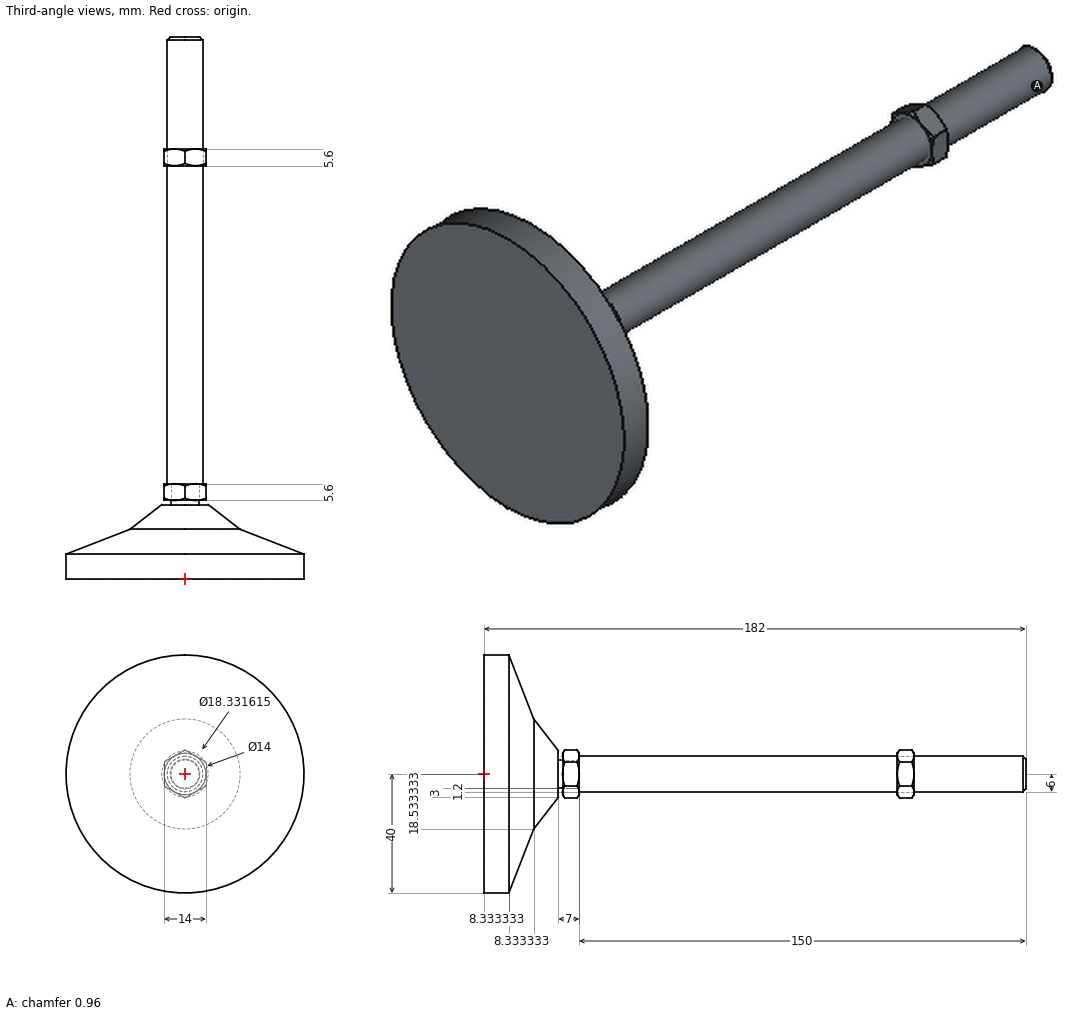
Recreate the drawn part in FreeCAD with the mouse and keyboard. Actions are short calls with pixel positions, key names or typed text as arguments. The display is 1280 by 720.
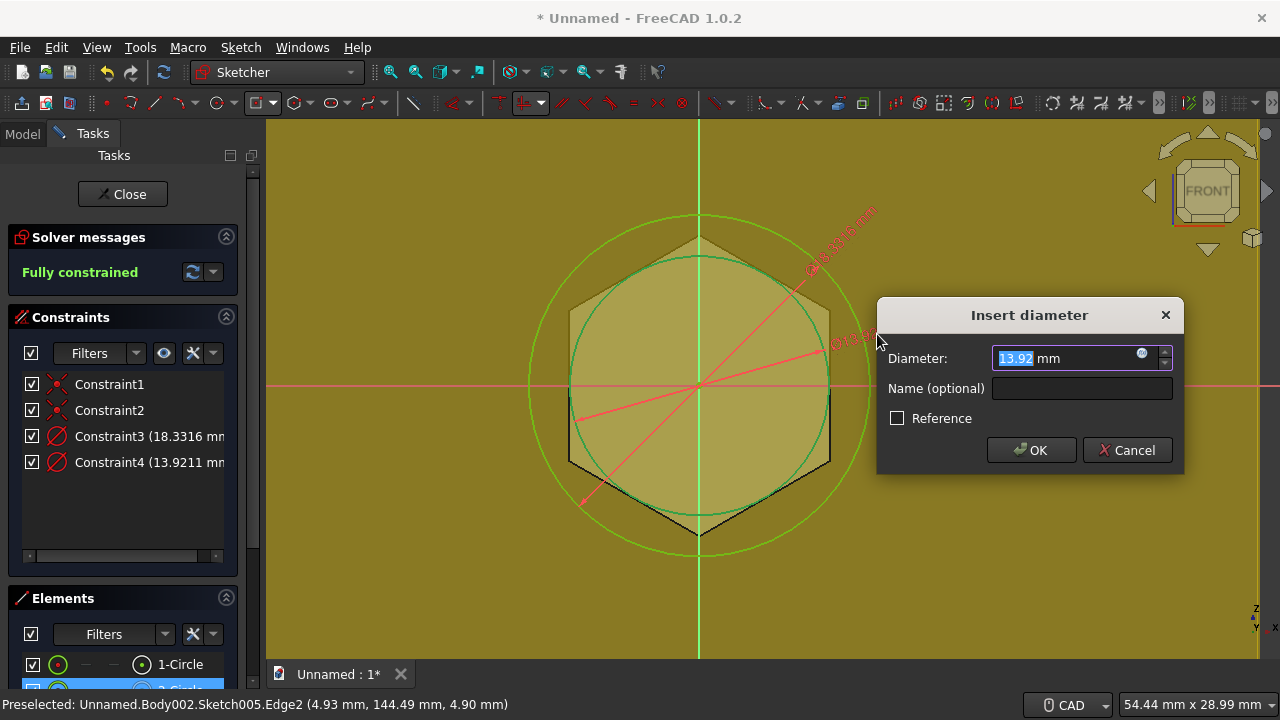
text(14)
key(Return)
key(Escape)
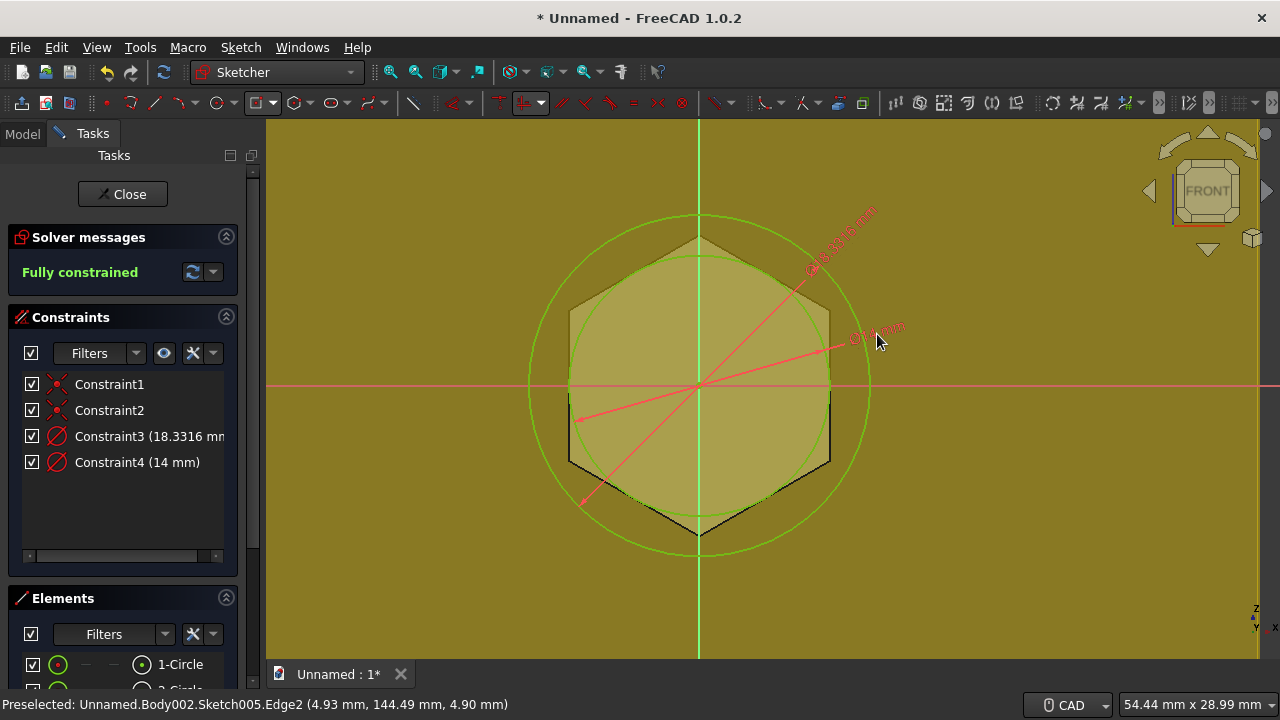
click(123, 194)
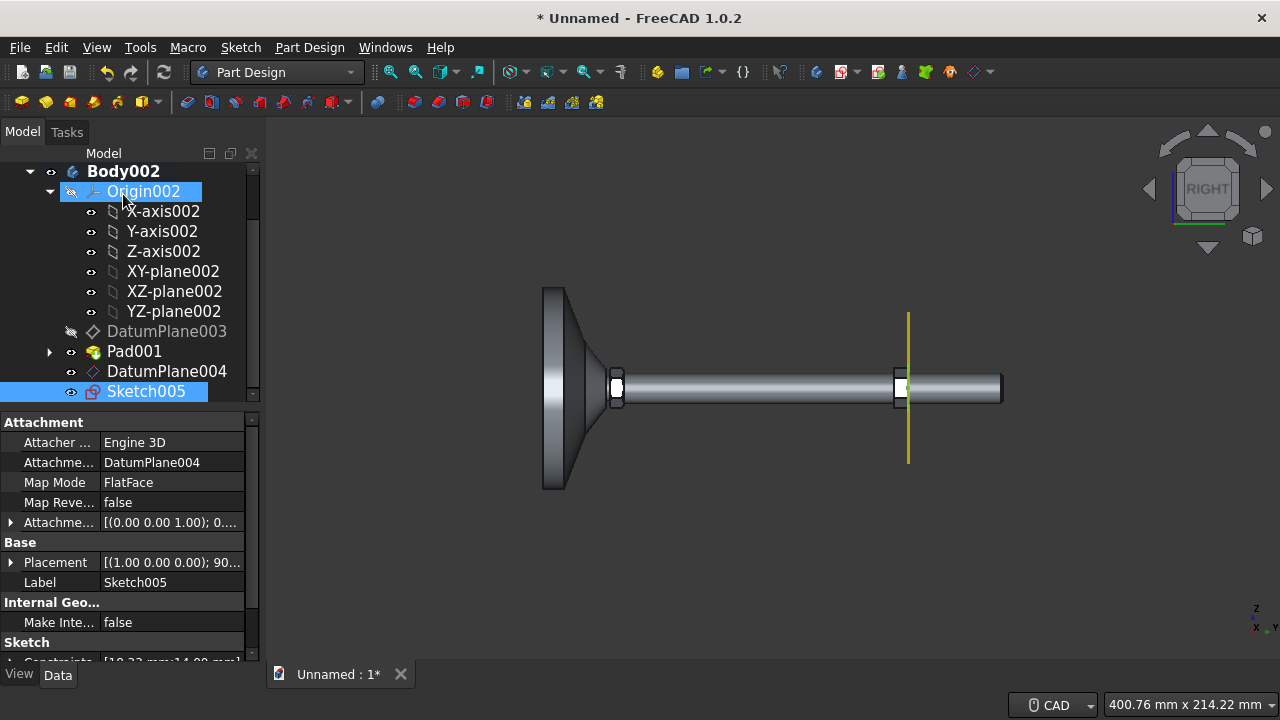
click(188, 102)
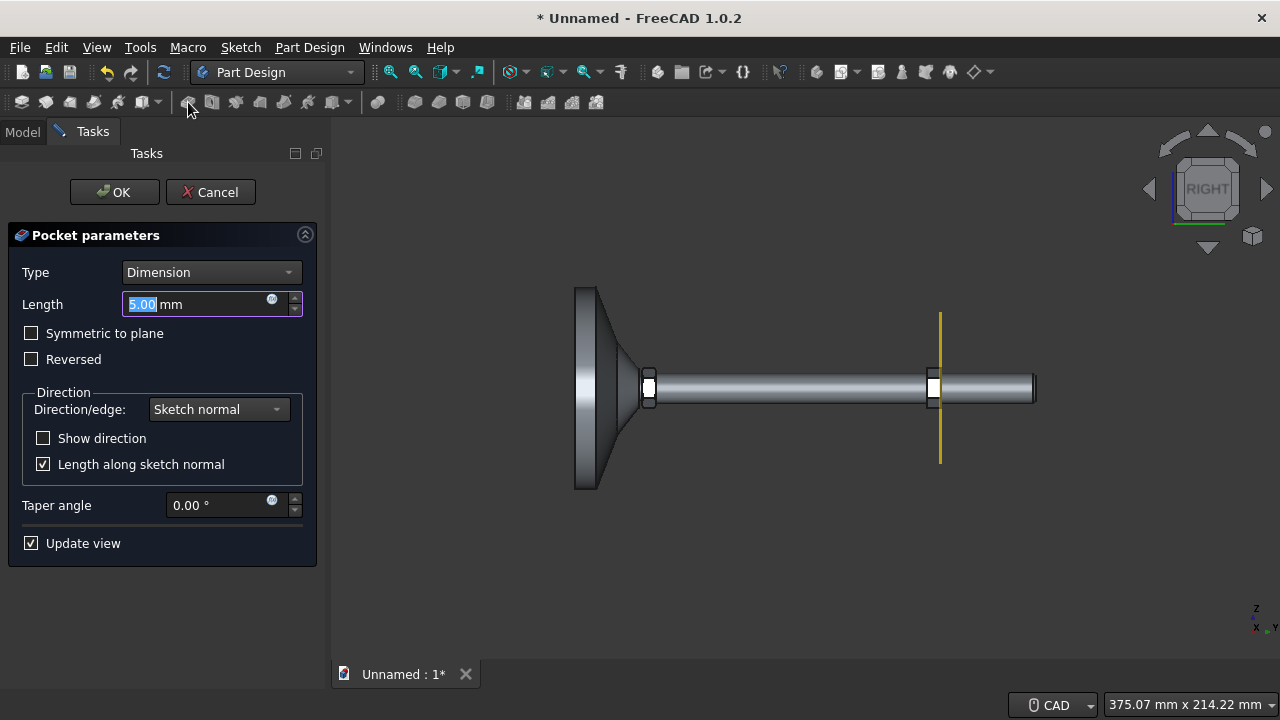
text(5.6)
key(Tab)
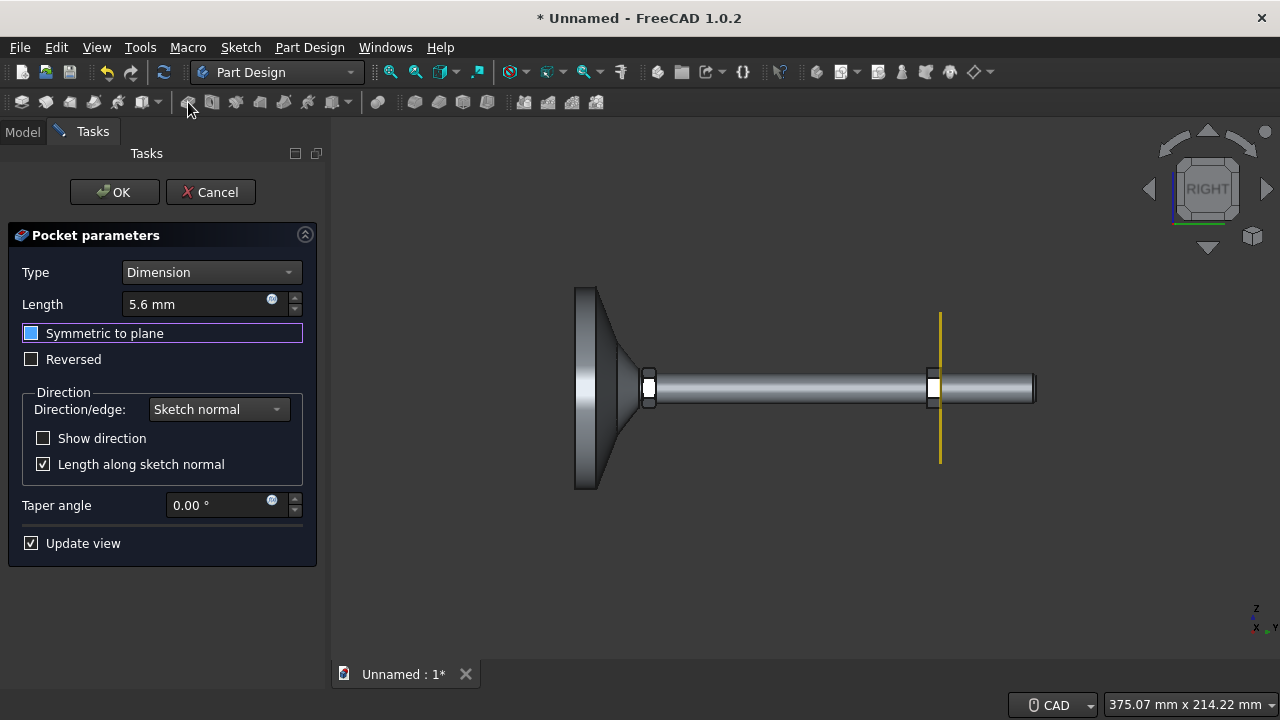
click(30, 359)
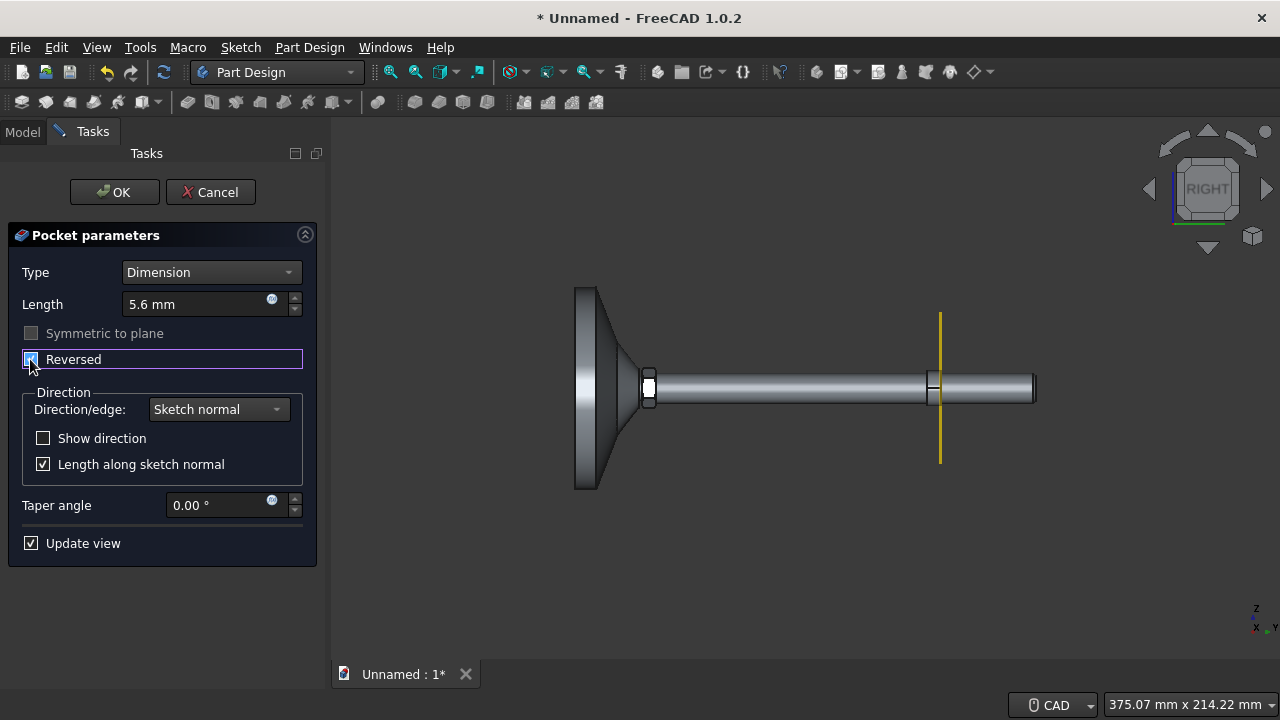
triple_click(226, 505)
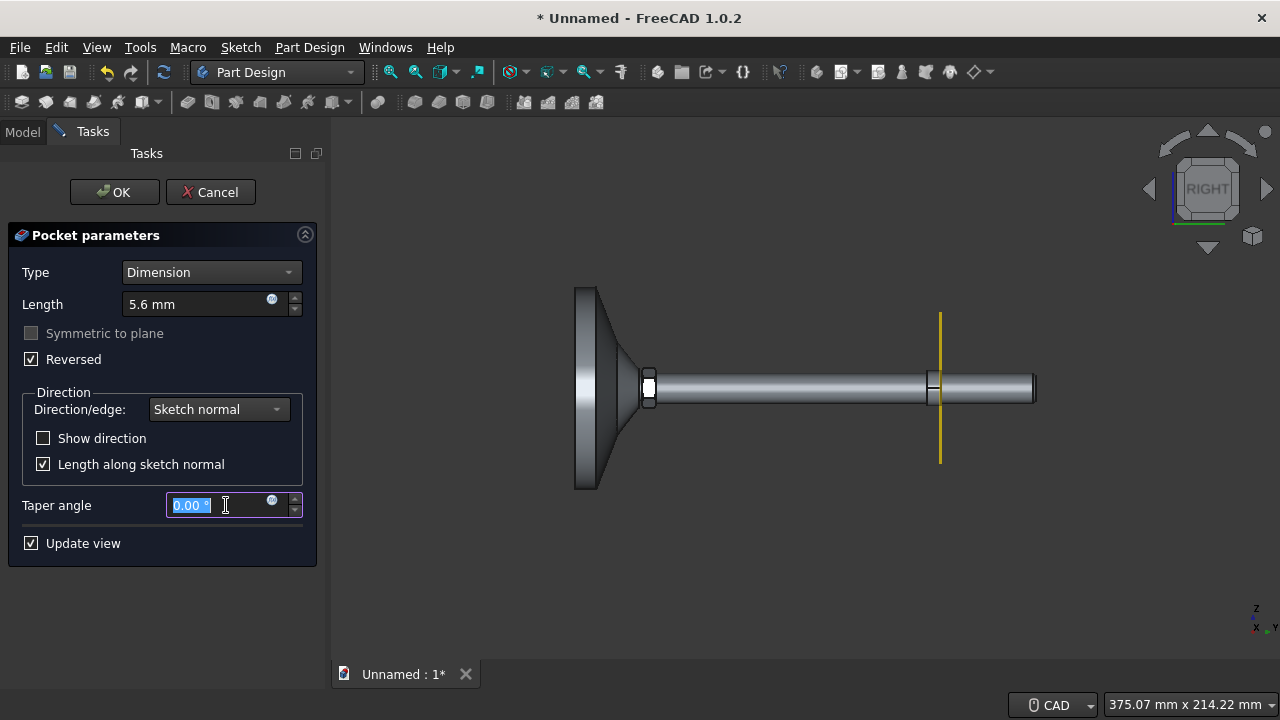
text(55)
key(Tab)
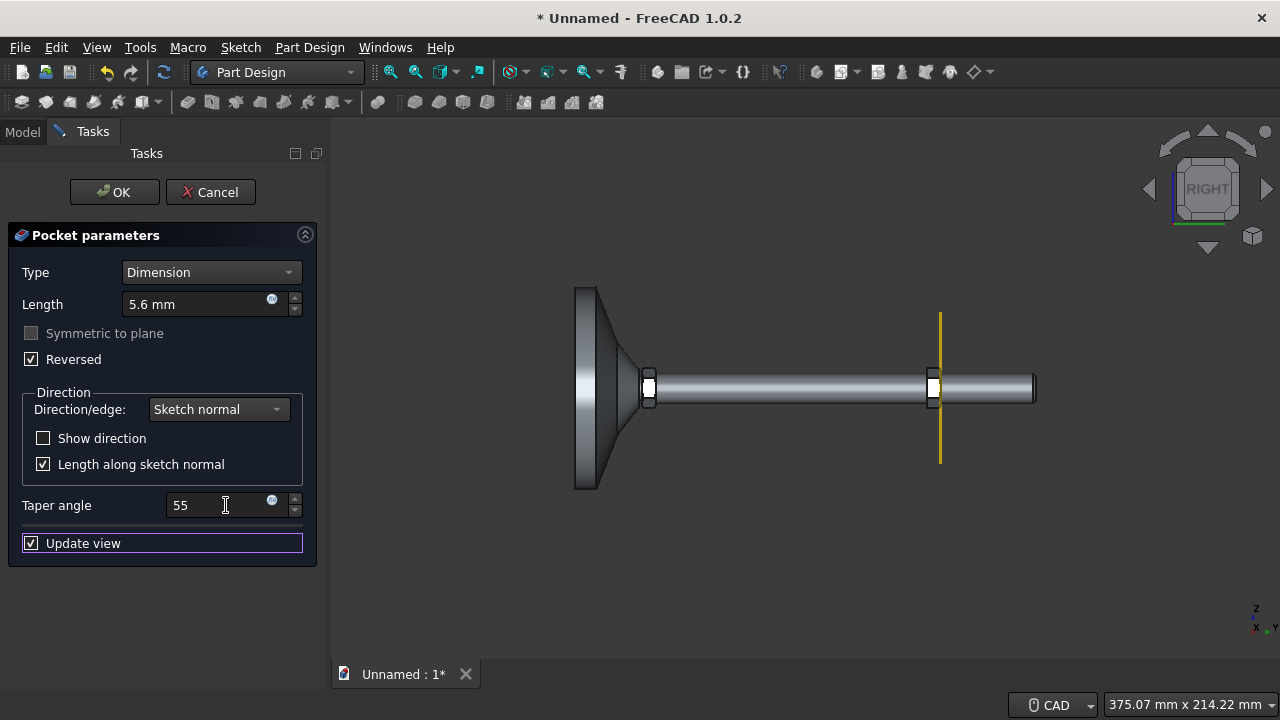
click(115, 192)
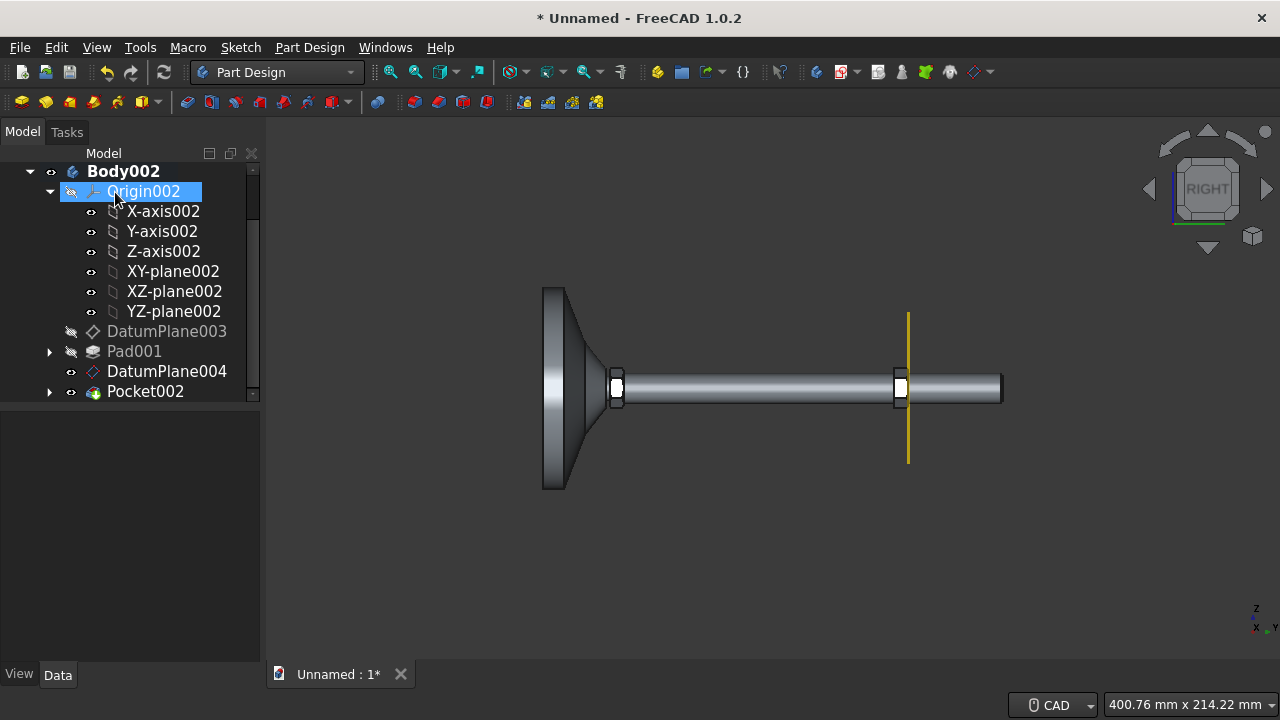
click(116, 372)
key(space)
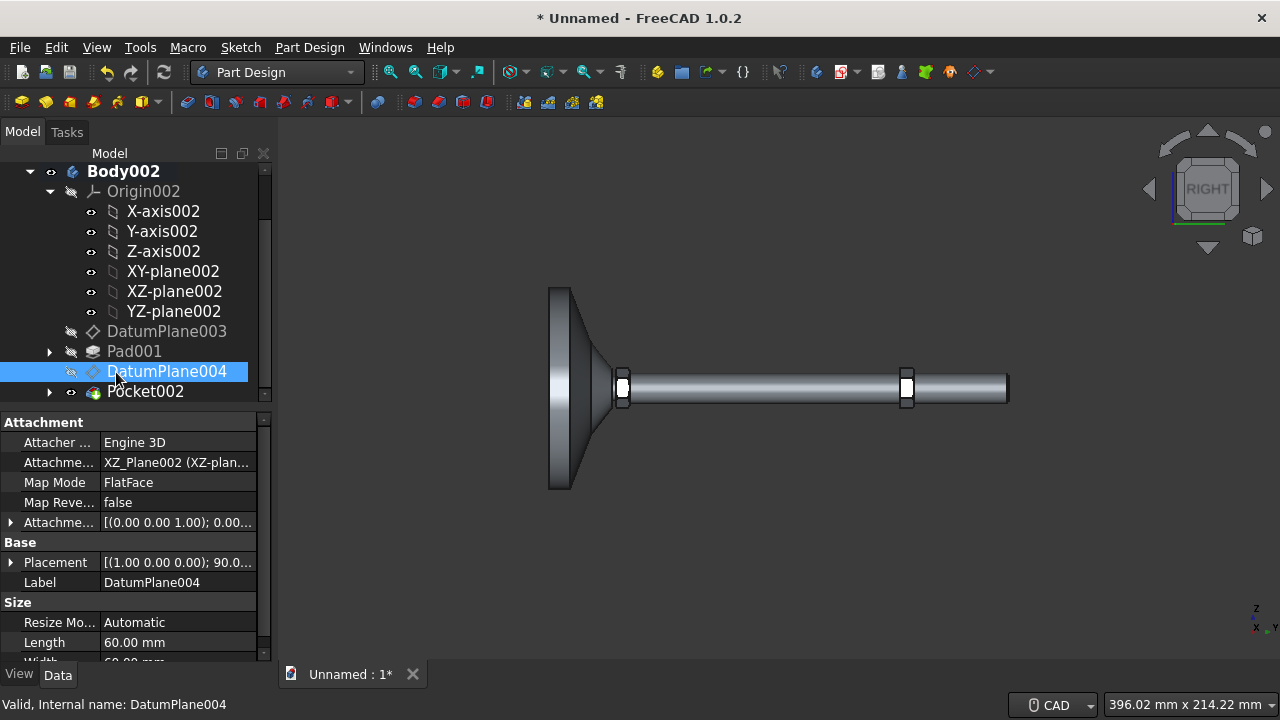
click(392, 72)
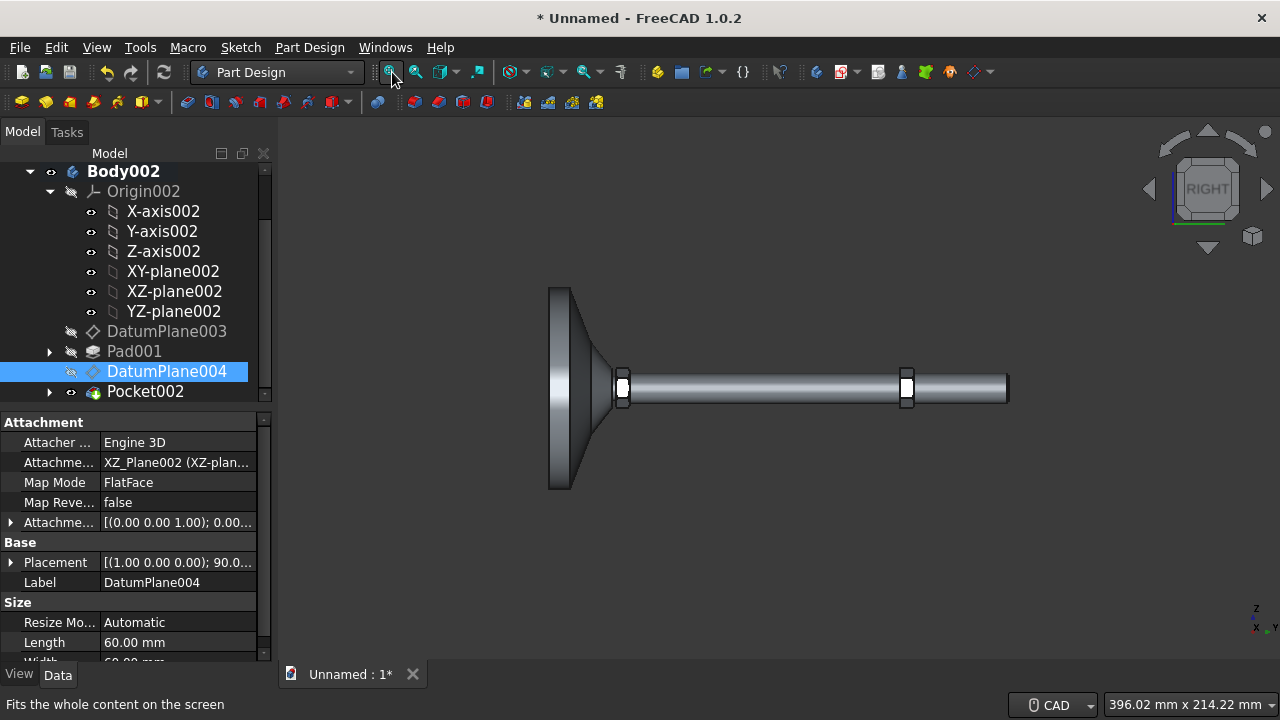
key(0)